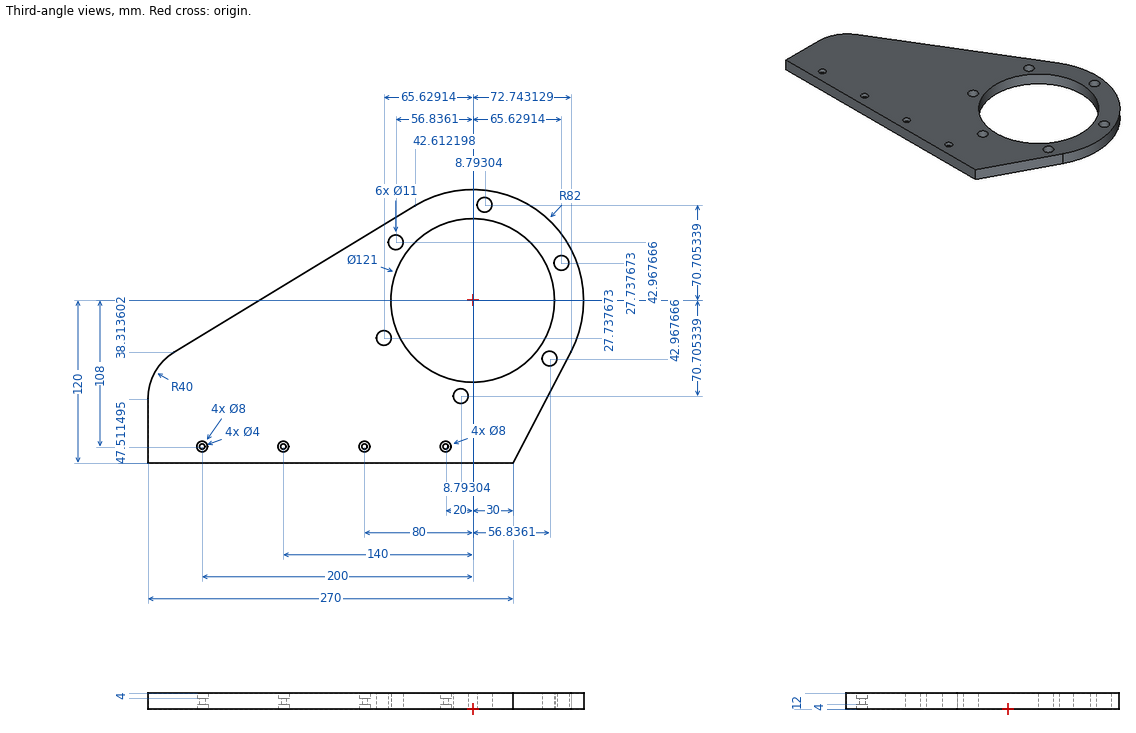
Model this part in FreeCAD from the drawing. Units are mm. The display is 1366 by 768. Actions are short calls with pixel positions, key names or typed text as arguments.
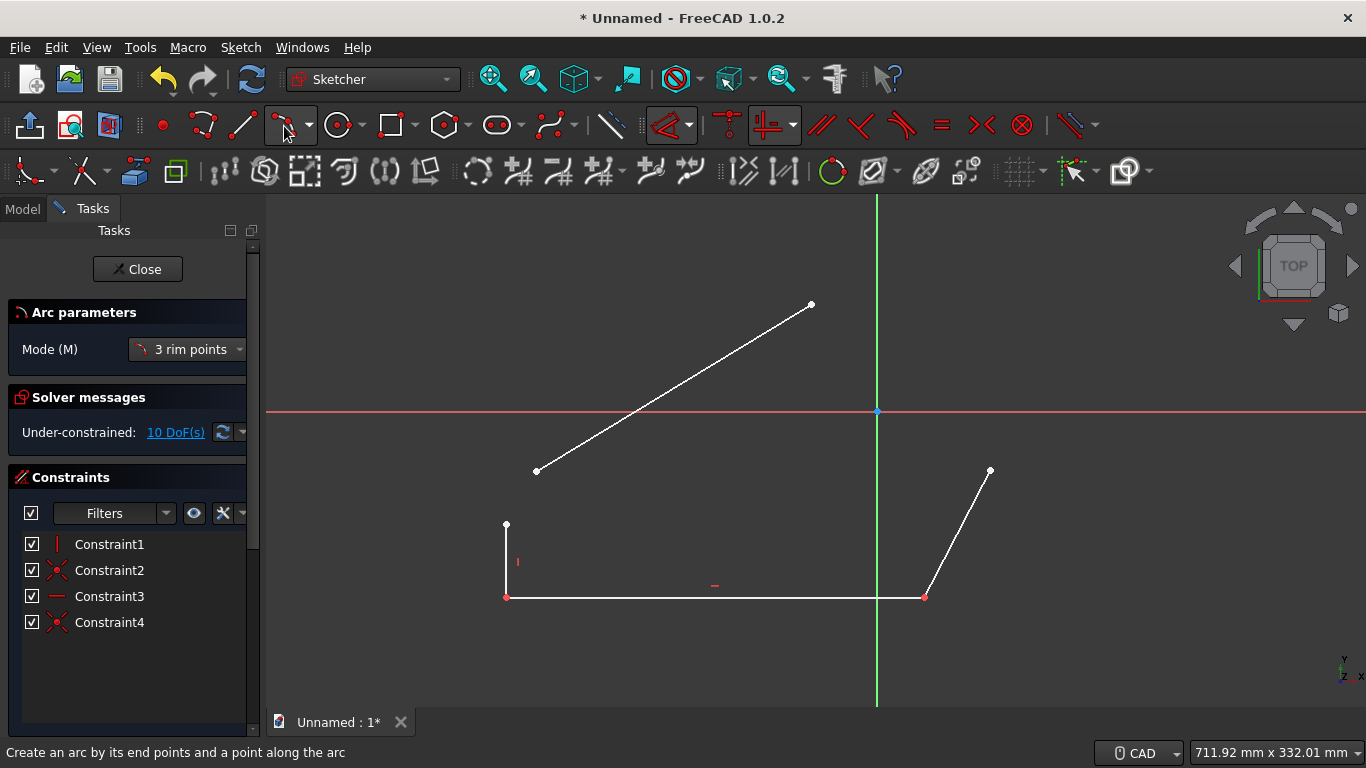
click(990, 471)
click(811, 305)
click(964, 319)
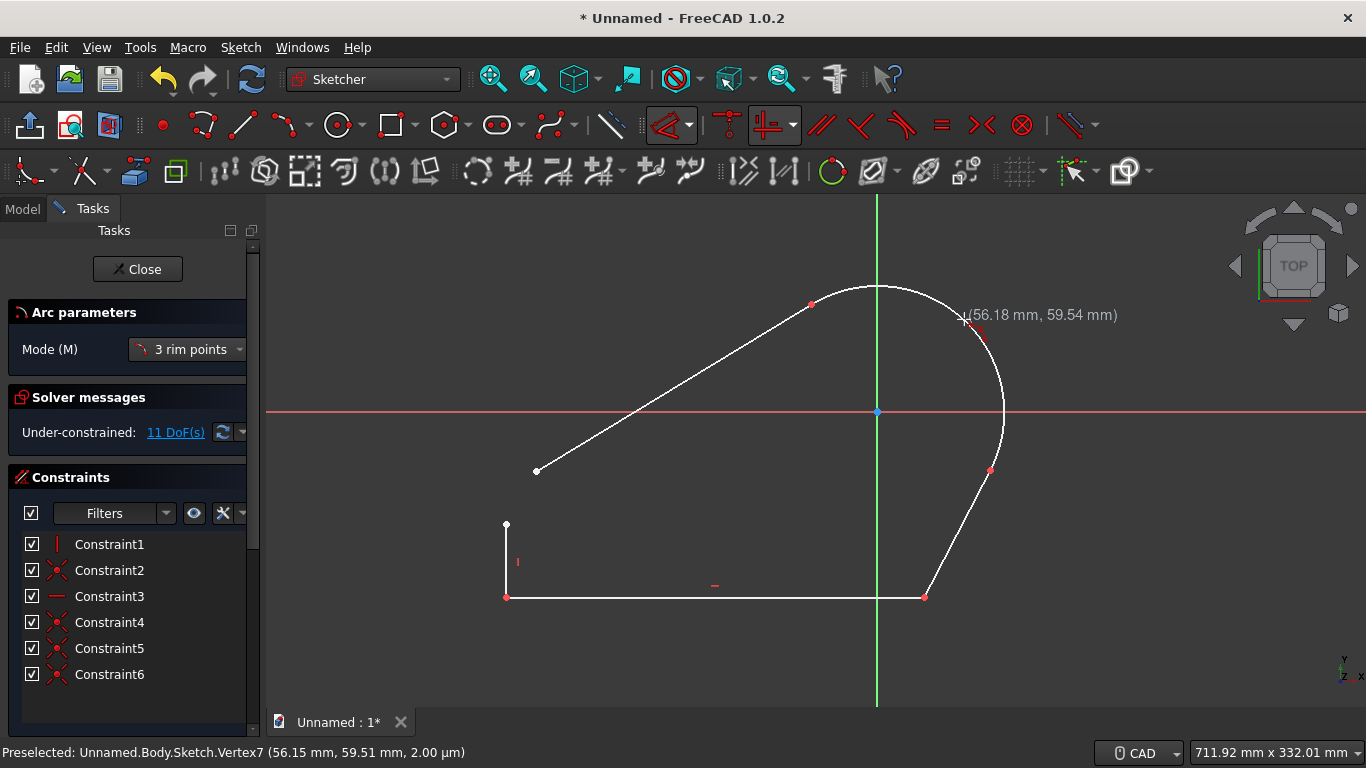
click(536, 472)
click(506, 525)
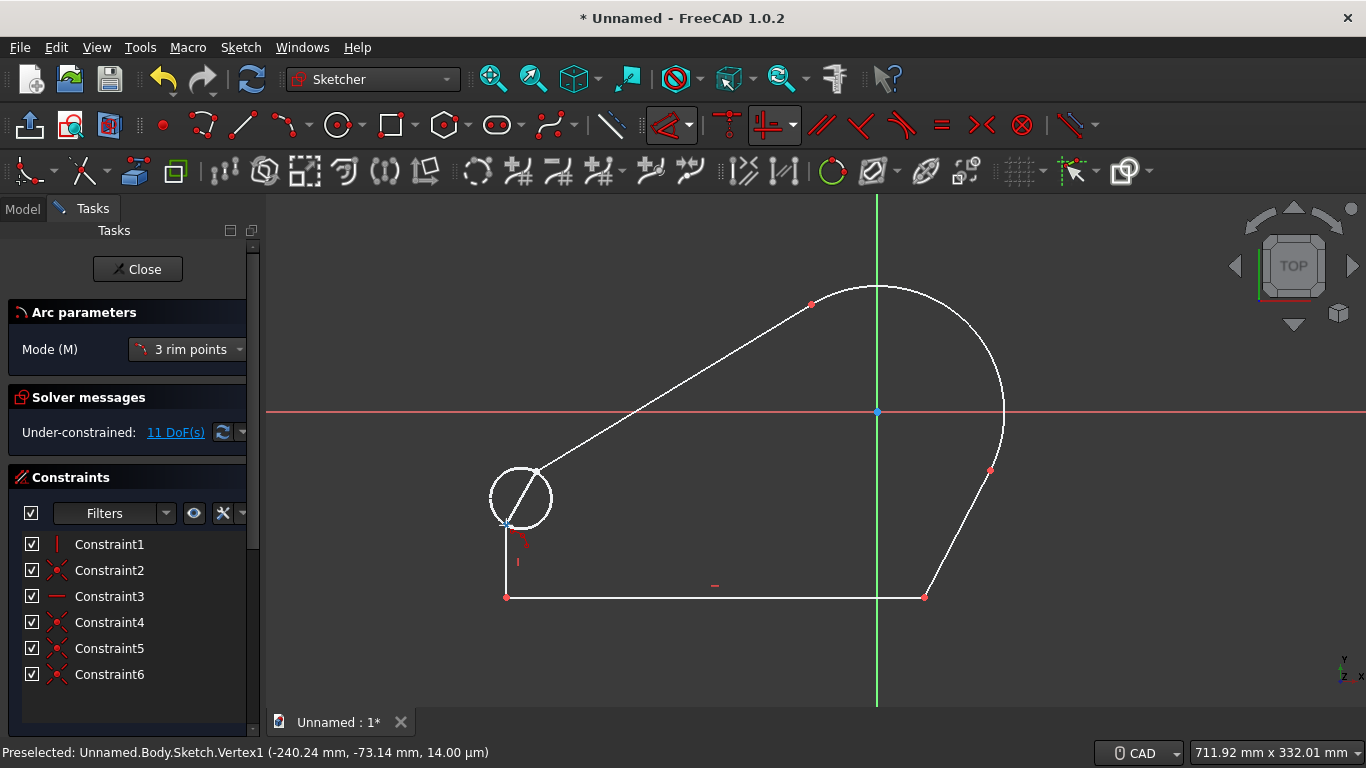
scroll(514, 494, up, 4)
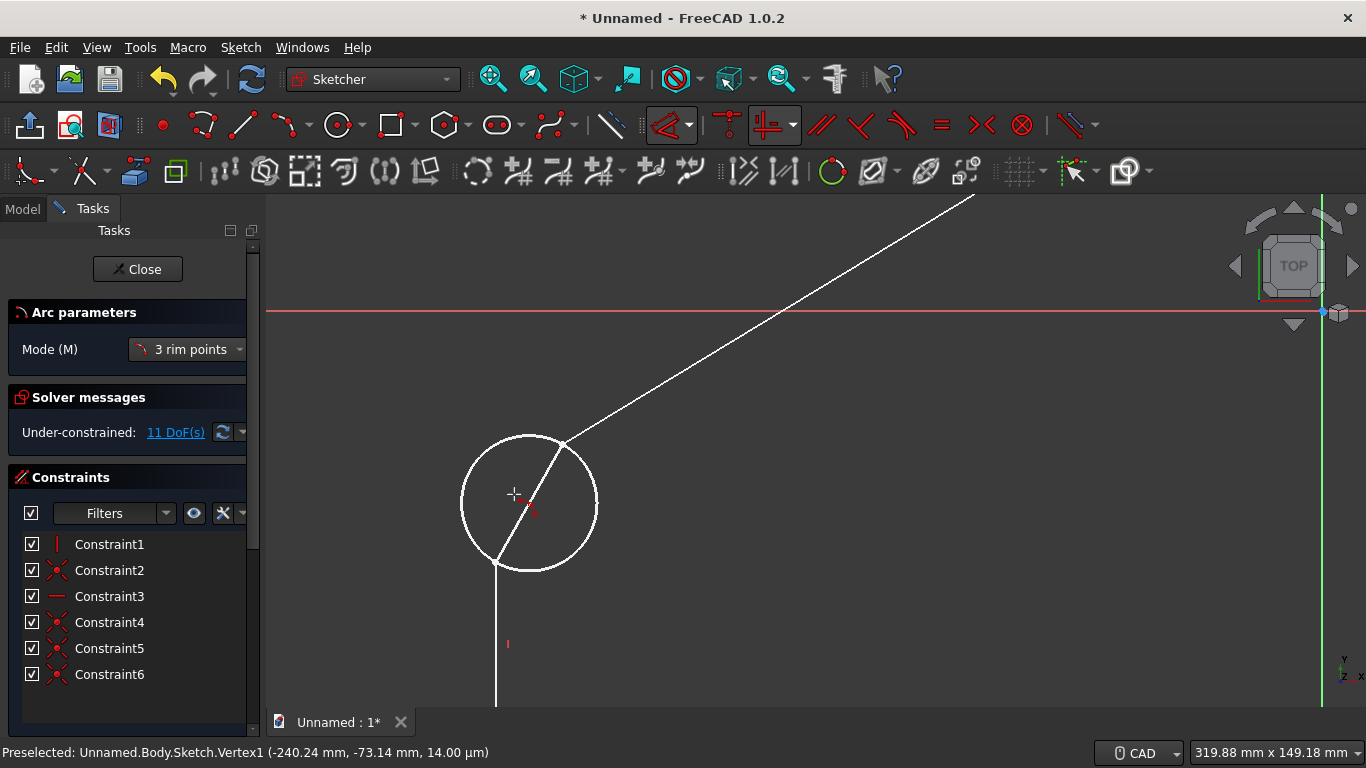
click(514, 493)
key(Escape)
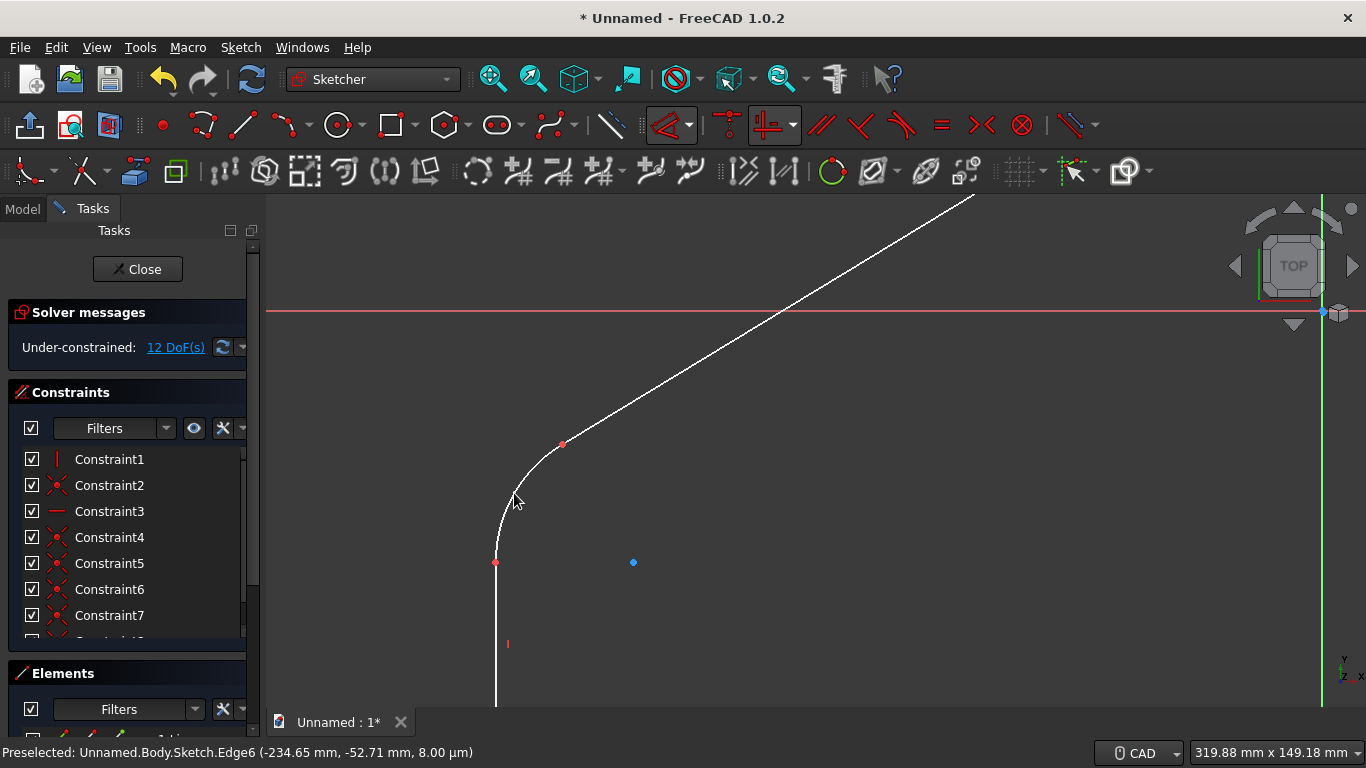
click(746, 333)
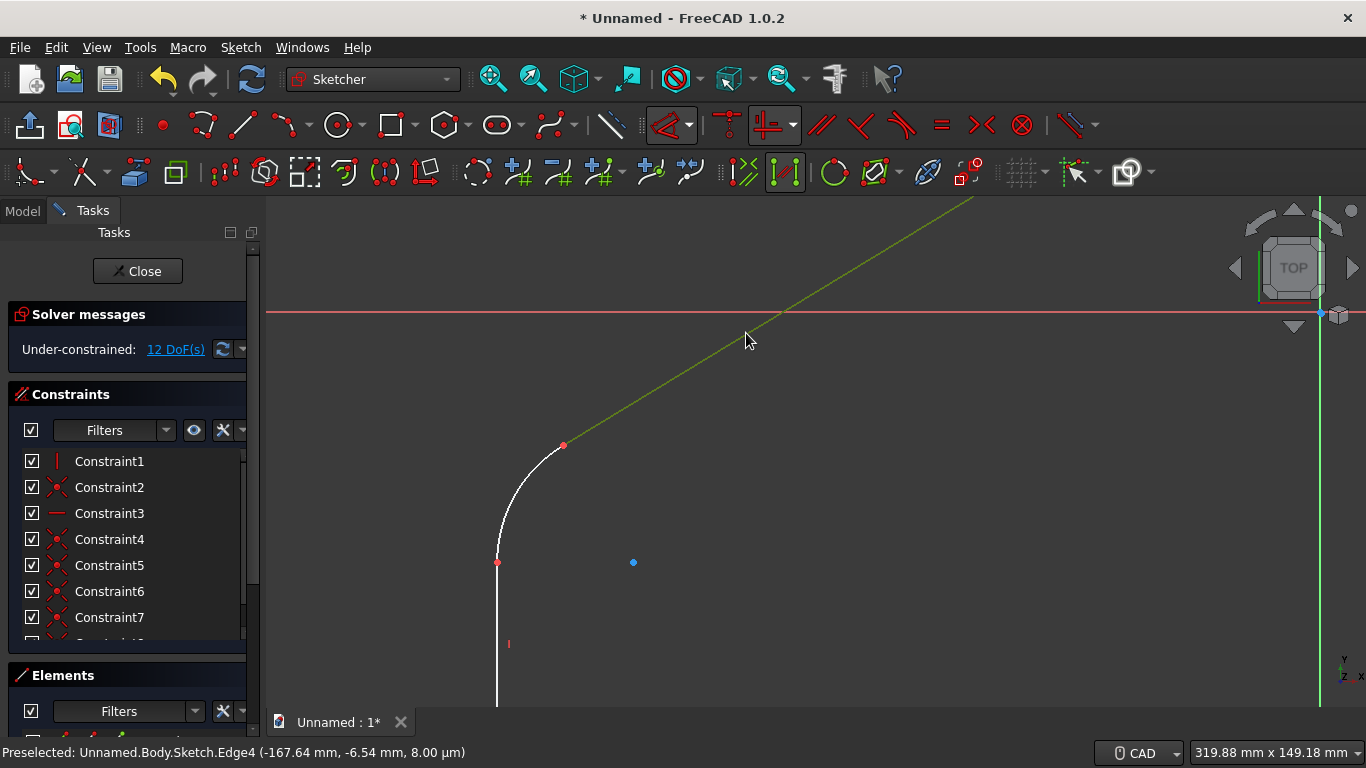
click(531, 472)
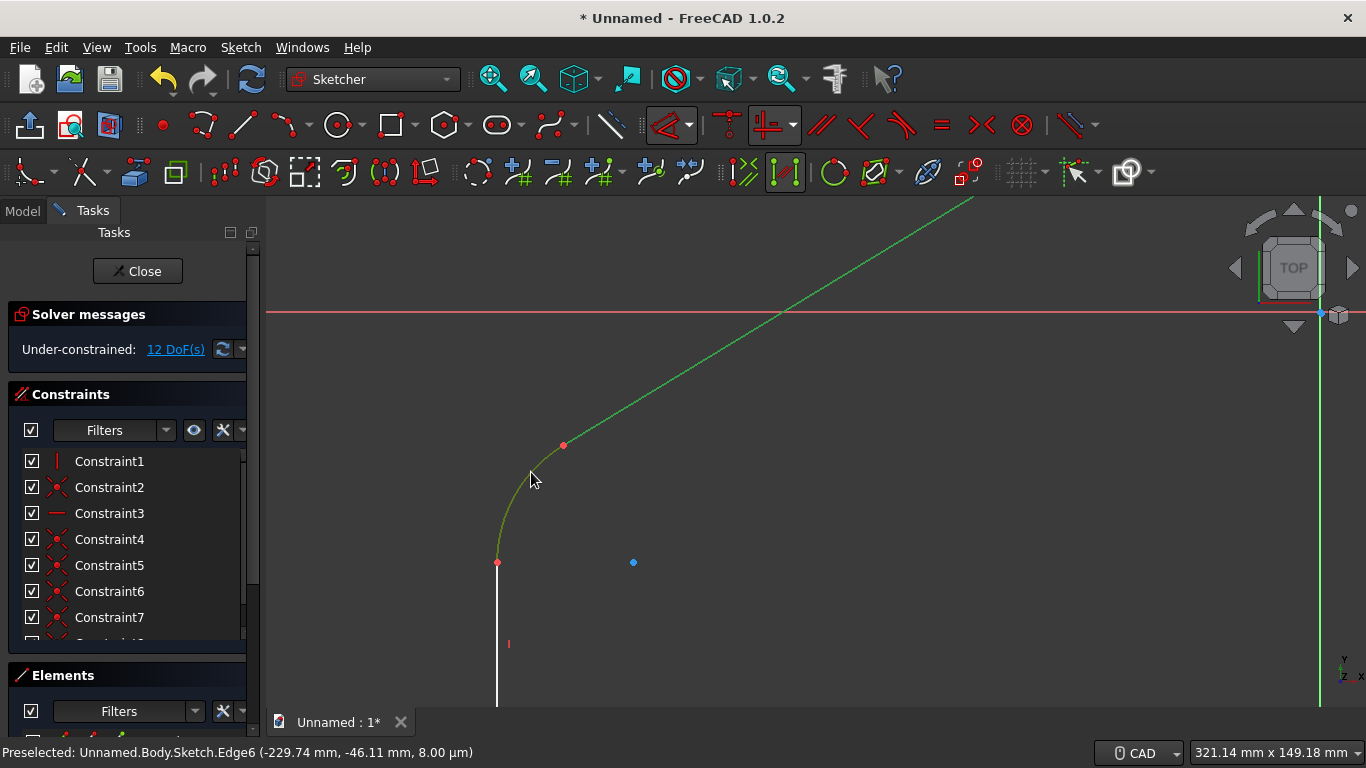
click(902, 126)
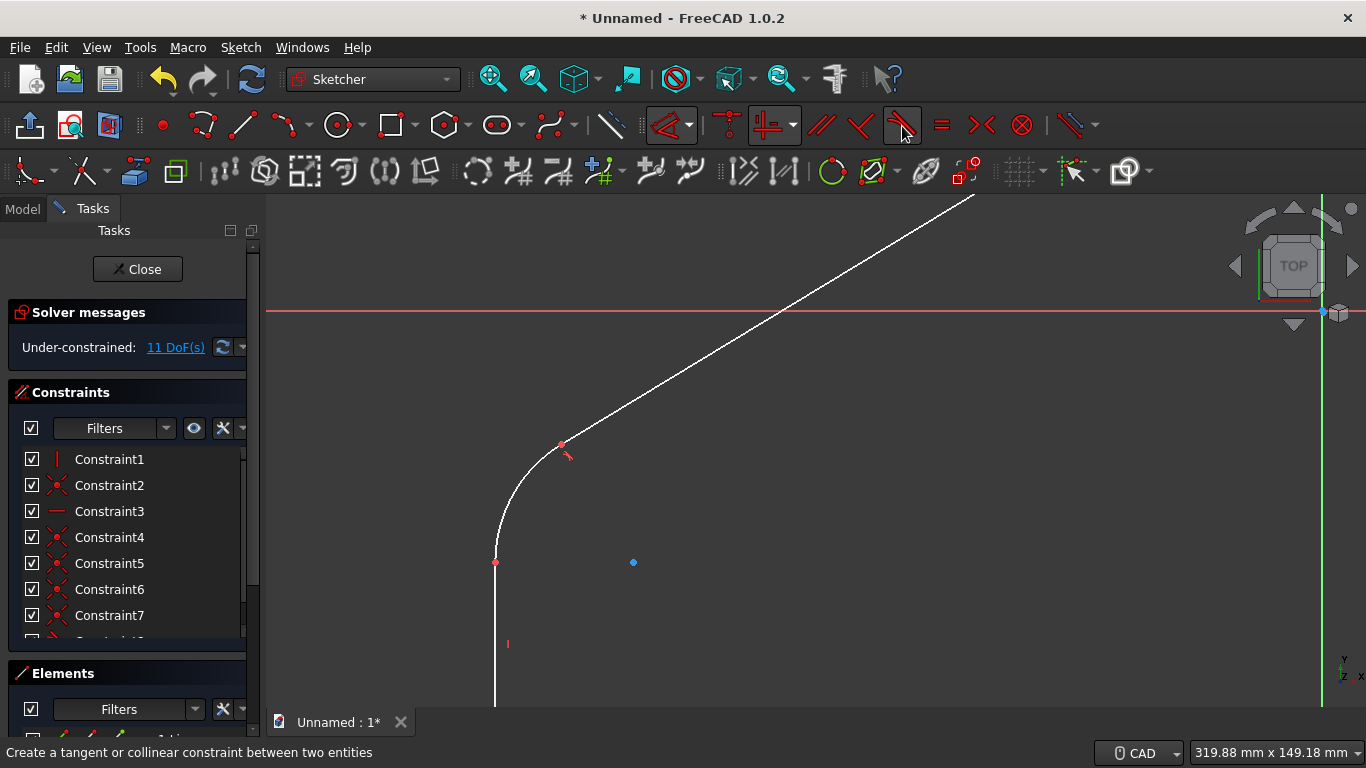
scroll(513, 494, down, 4)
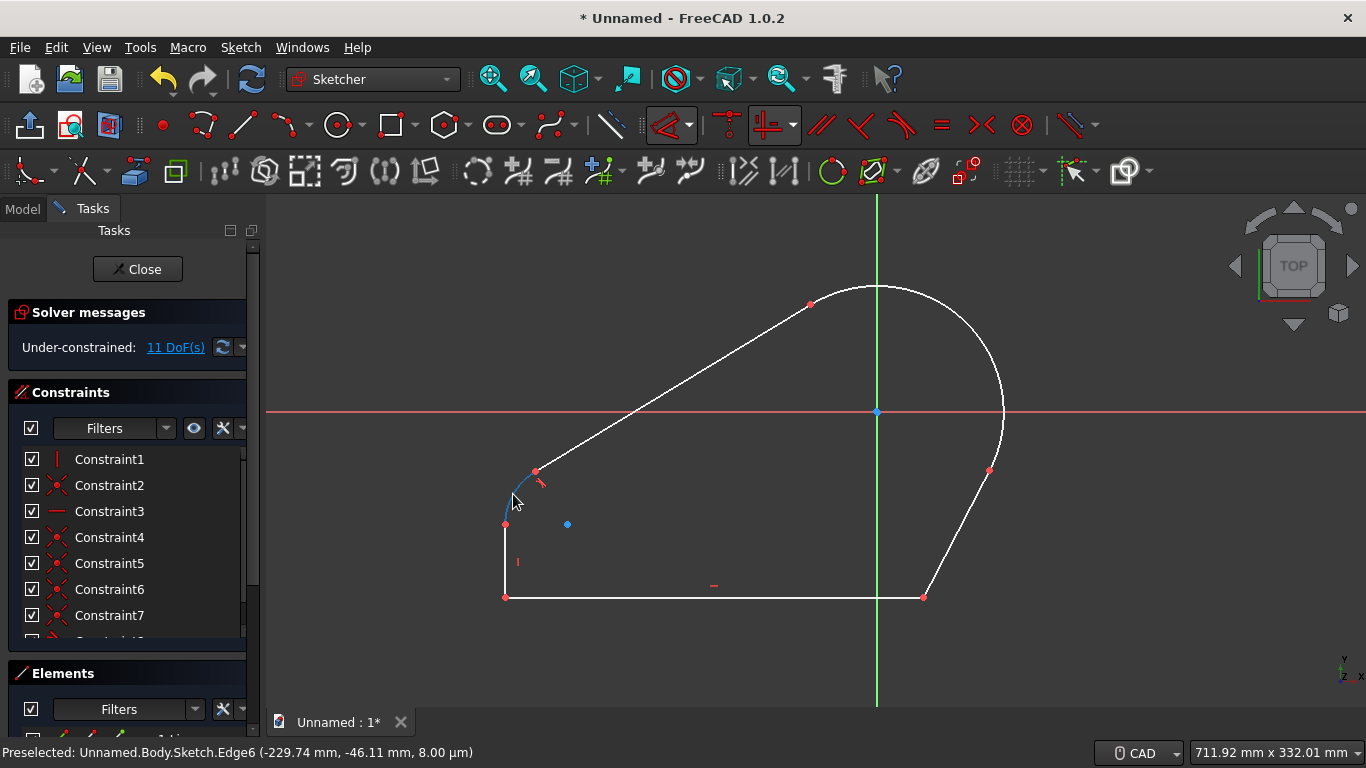
drag(867, 402, 887, 423)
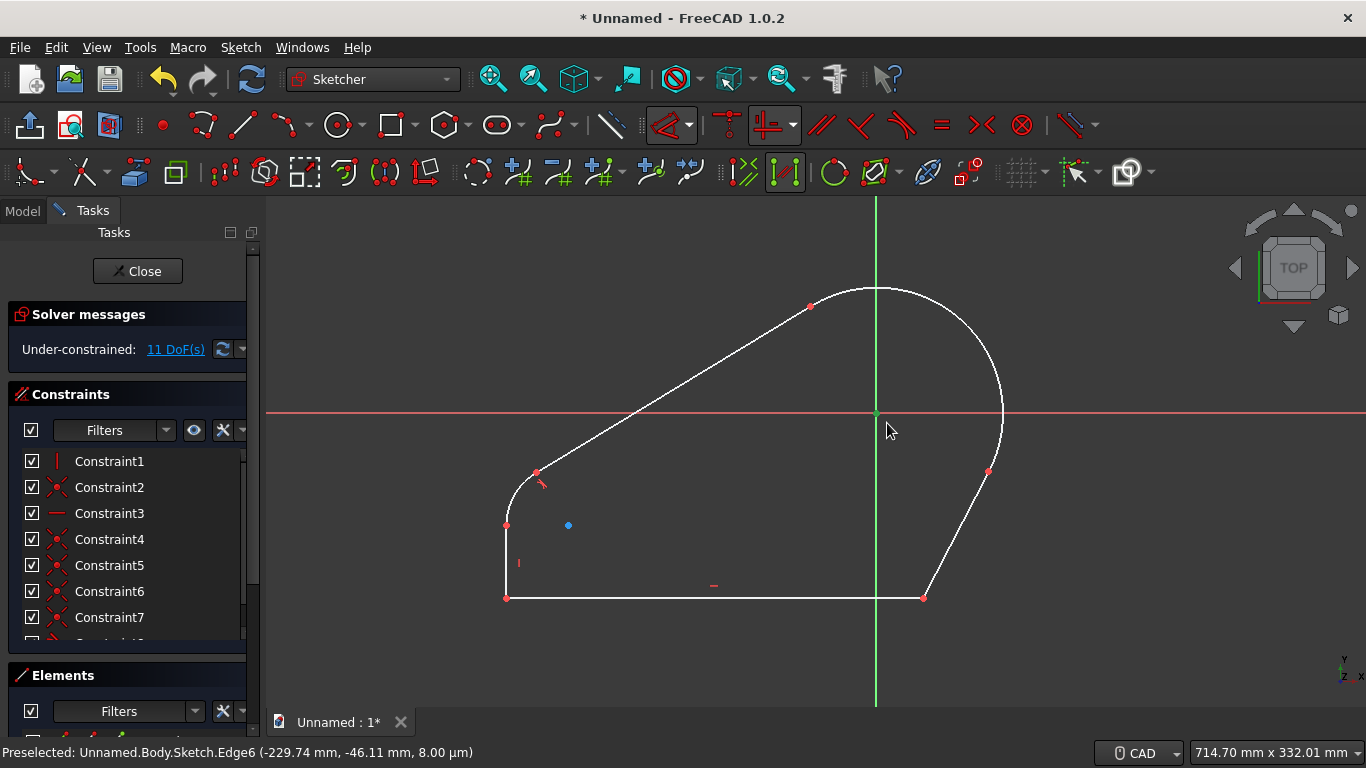
click(728, 126)